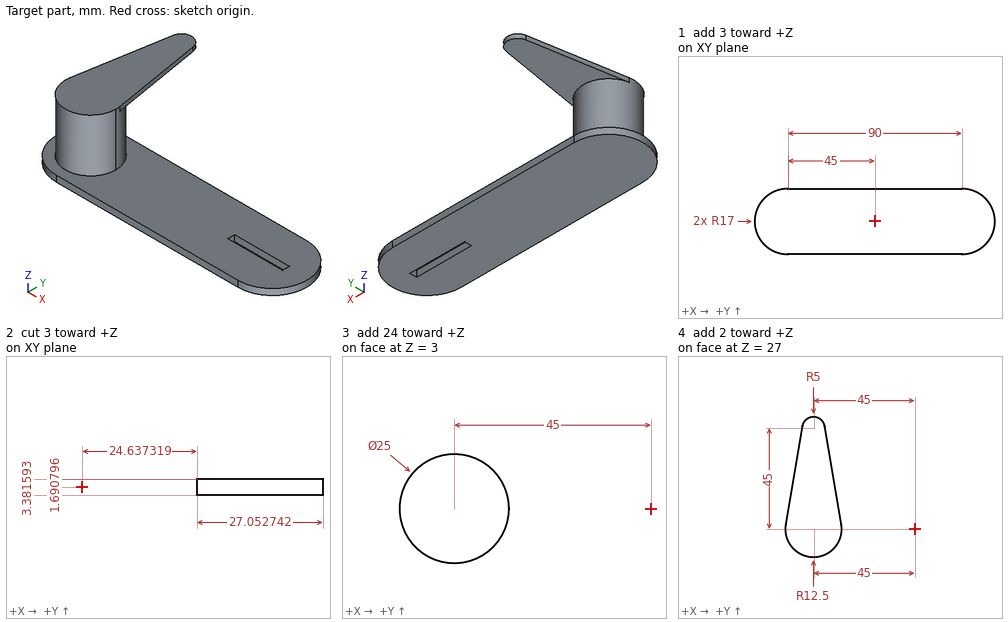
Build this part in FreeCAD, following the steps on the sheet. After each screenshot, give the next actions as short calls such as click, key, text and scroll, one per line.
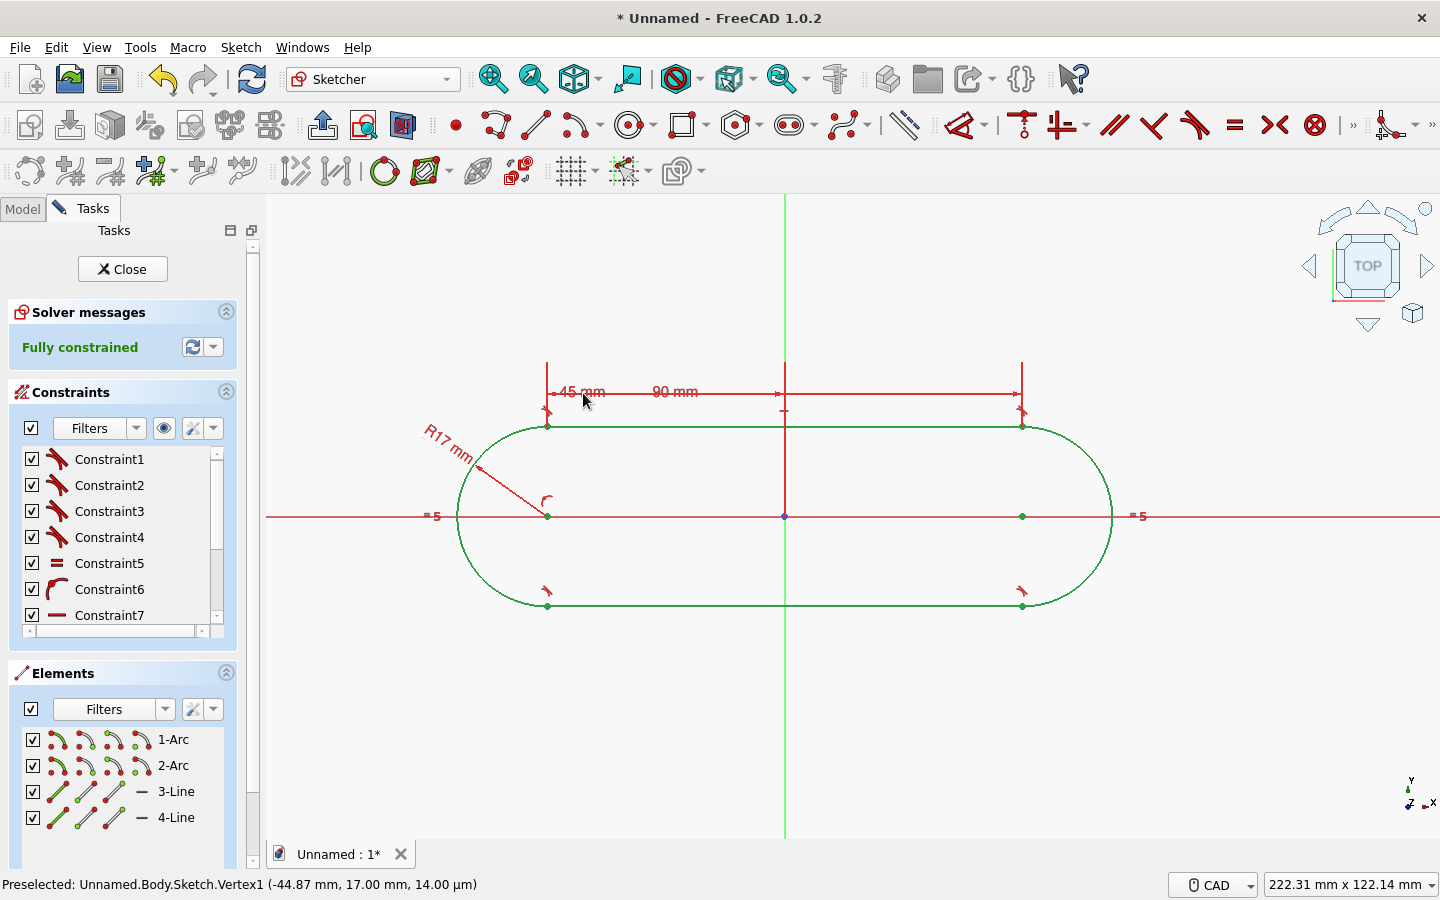
click(123, 269)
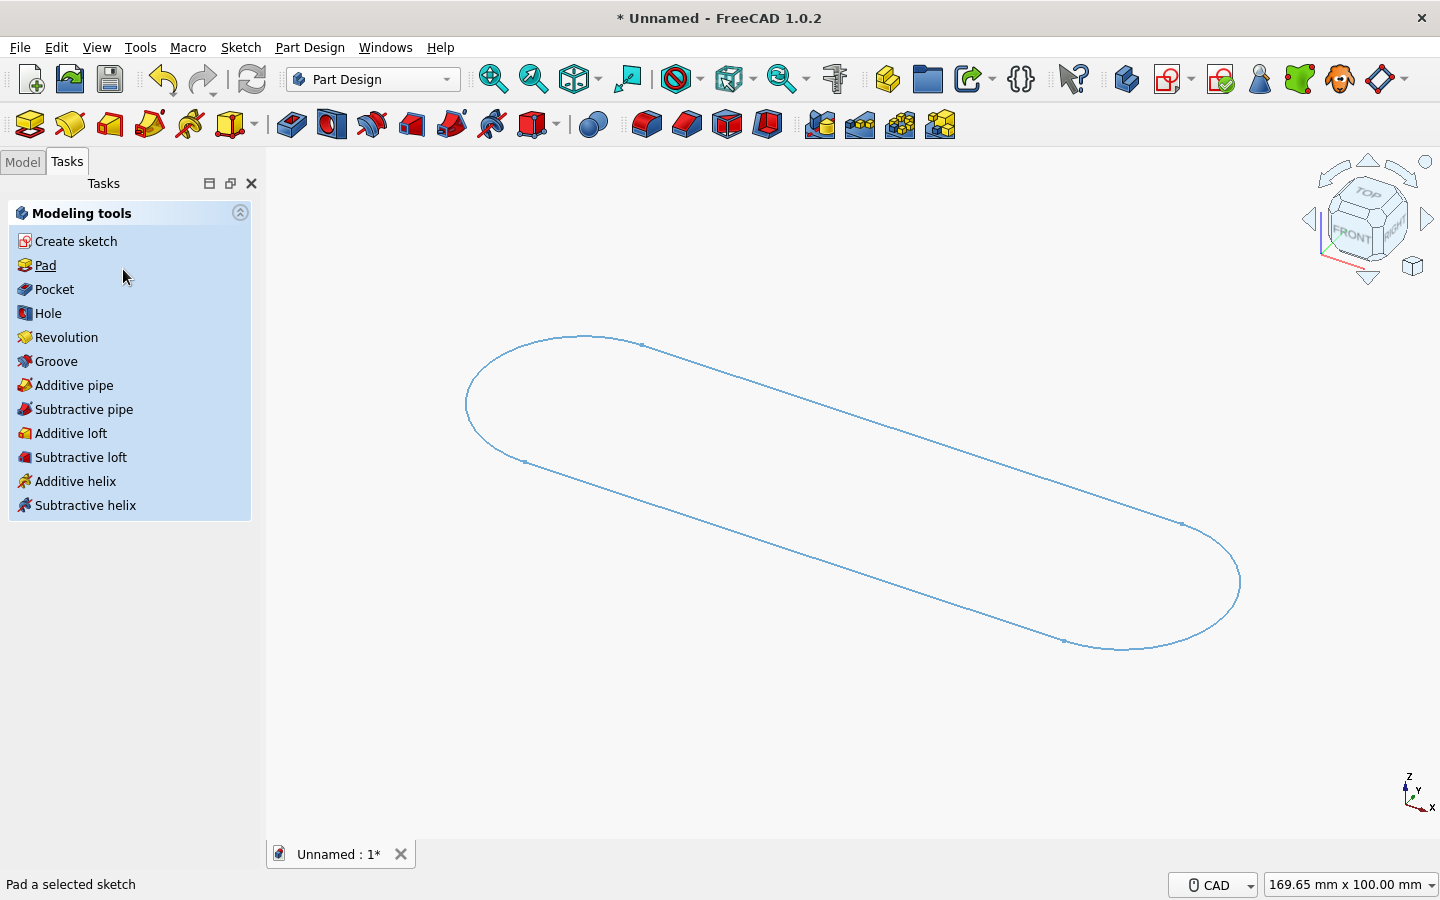
click(30, 124)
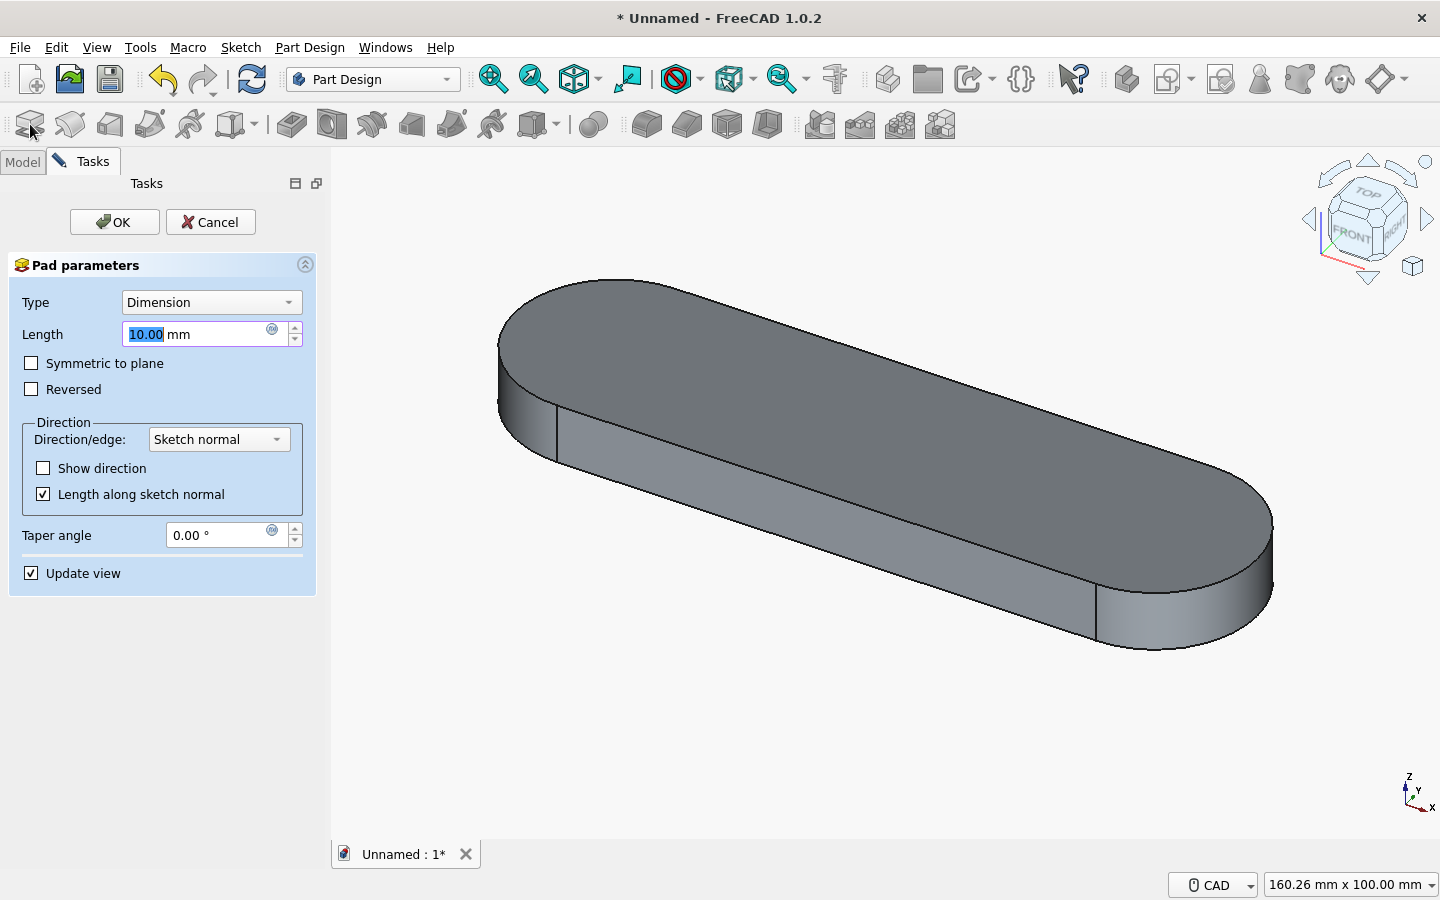
text(3)
key(Tab)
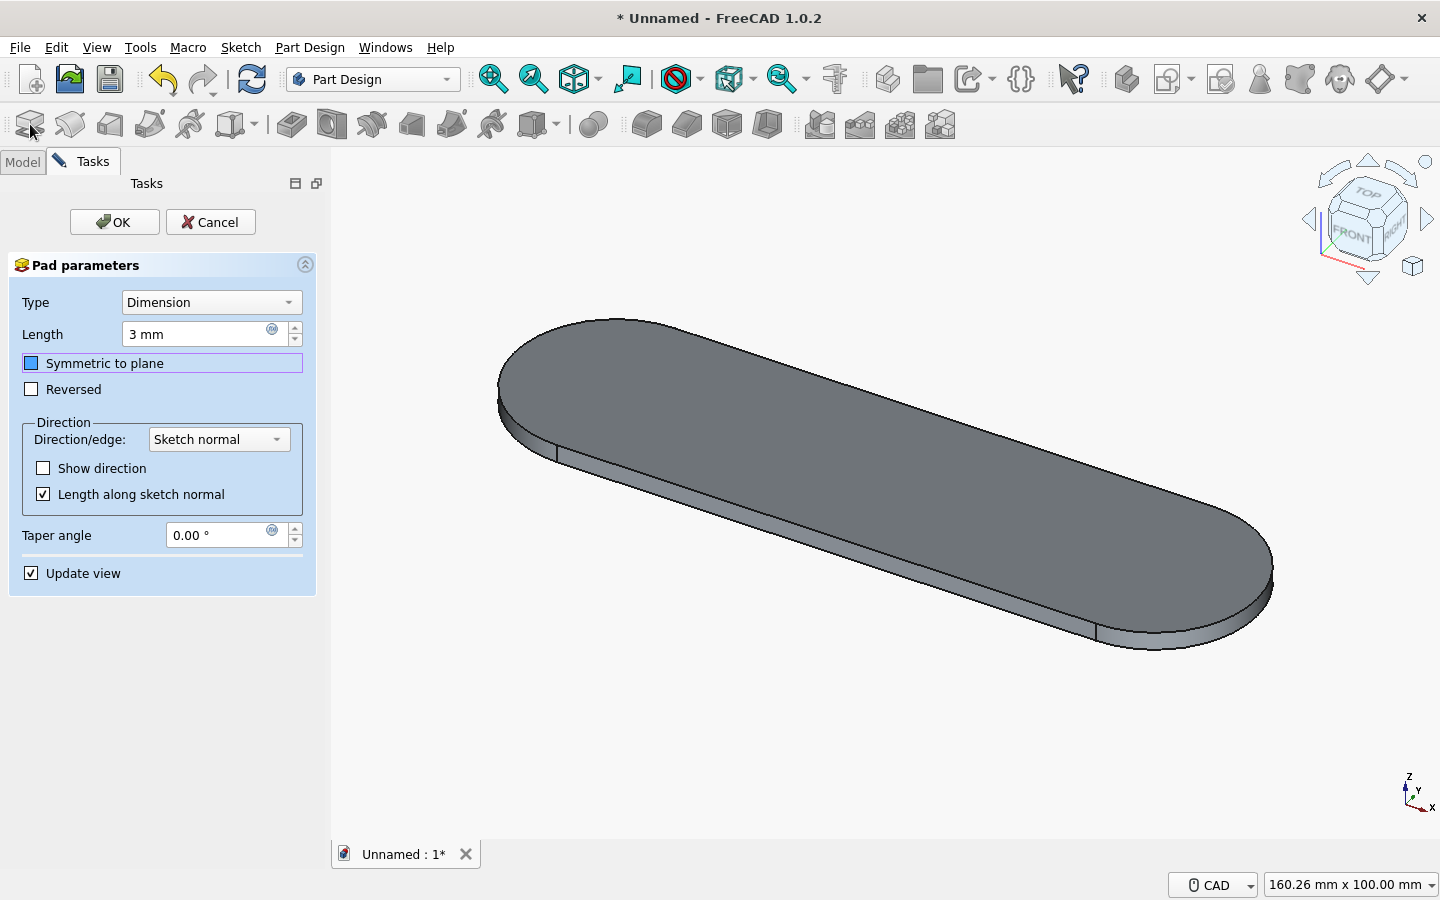
click(115, 222)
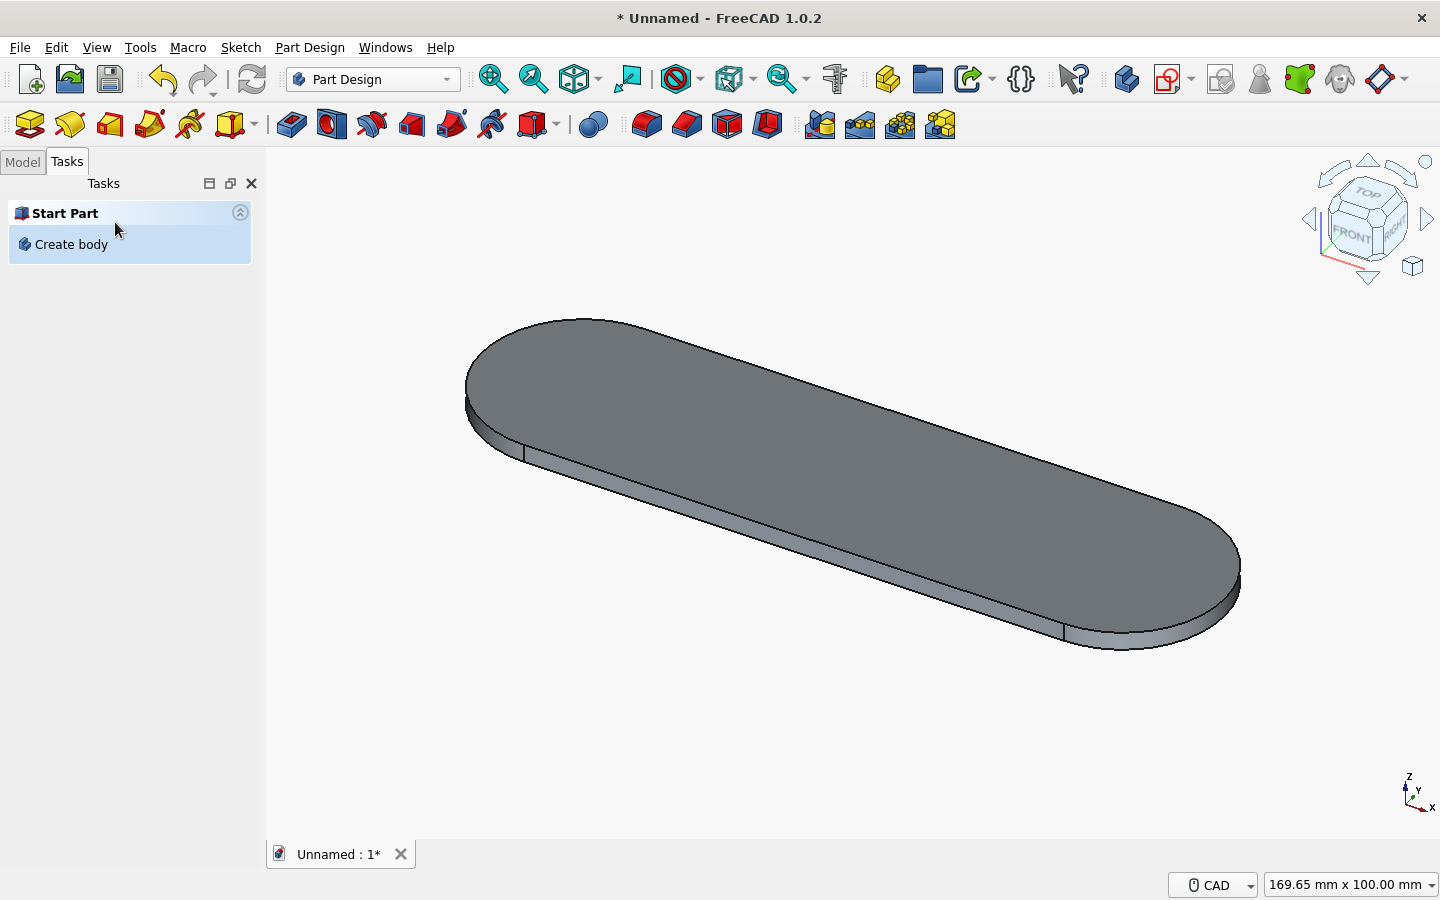
click(1168, 80)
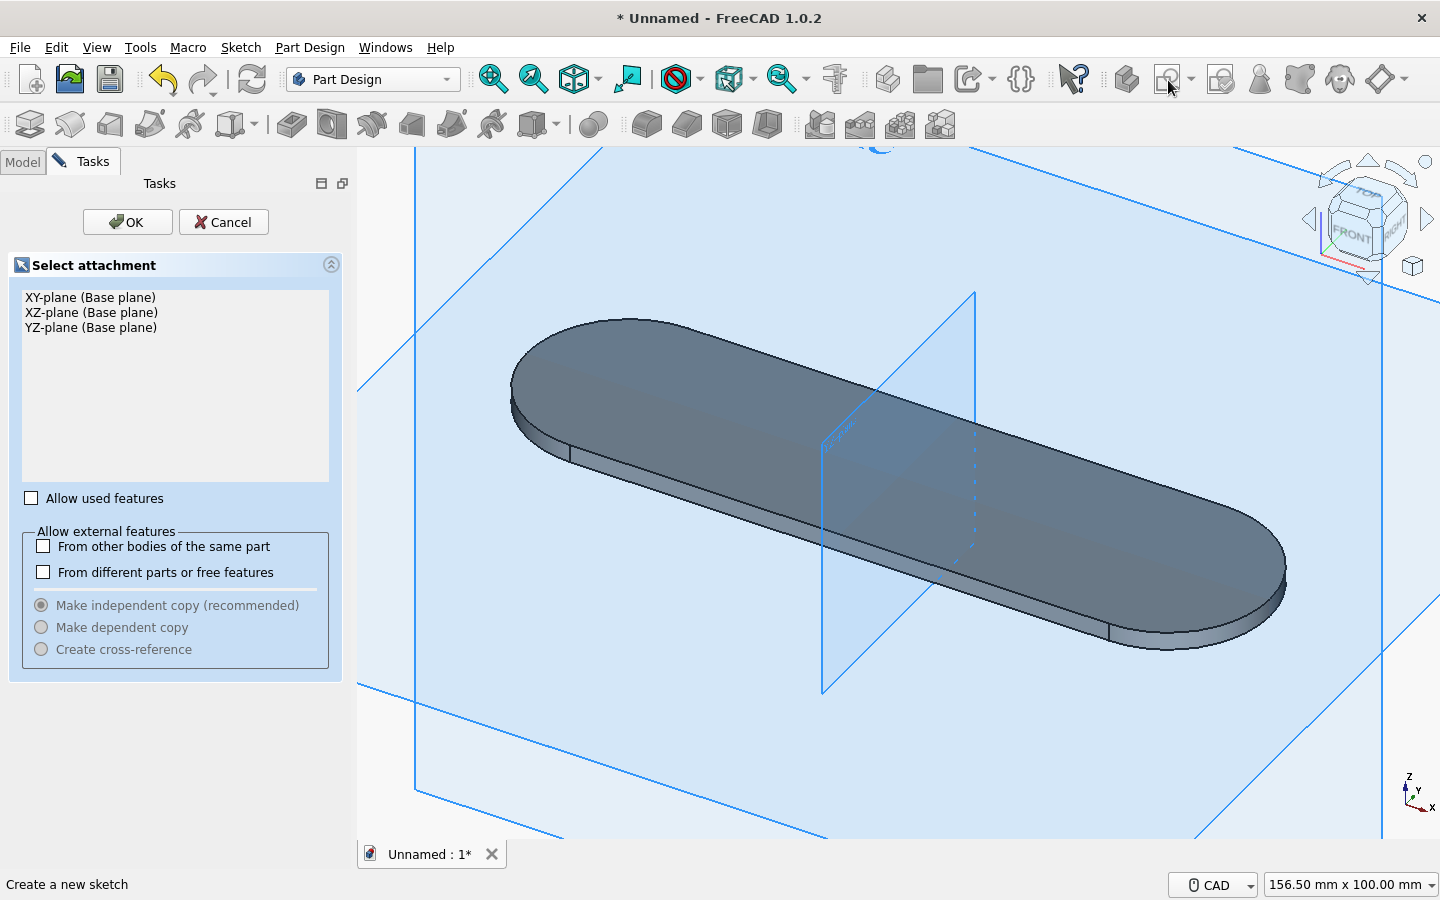
click(82, 298)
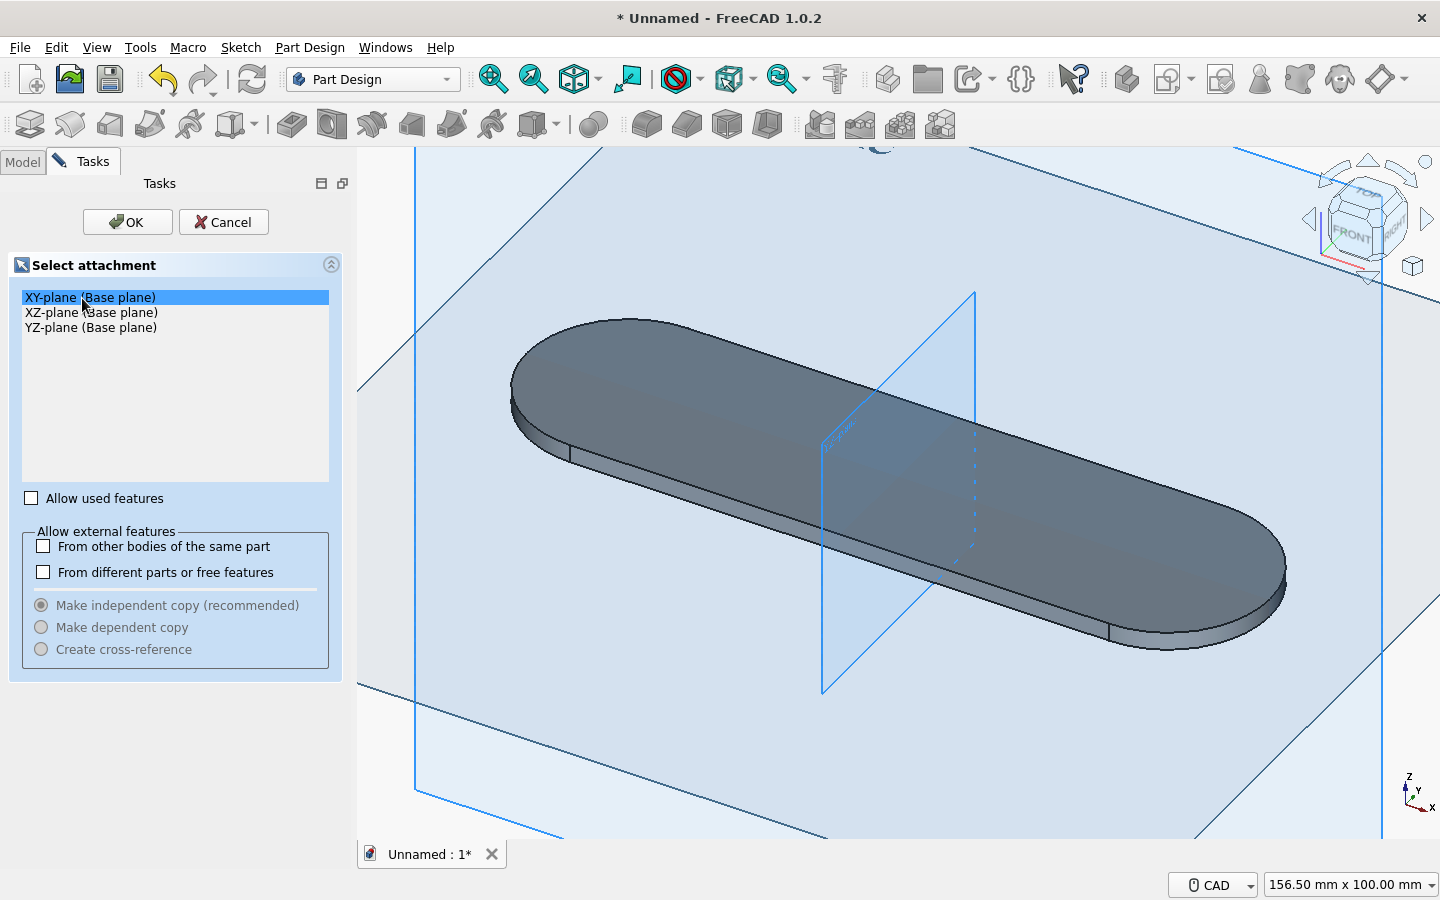
click(128, 222)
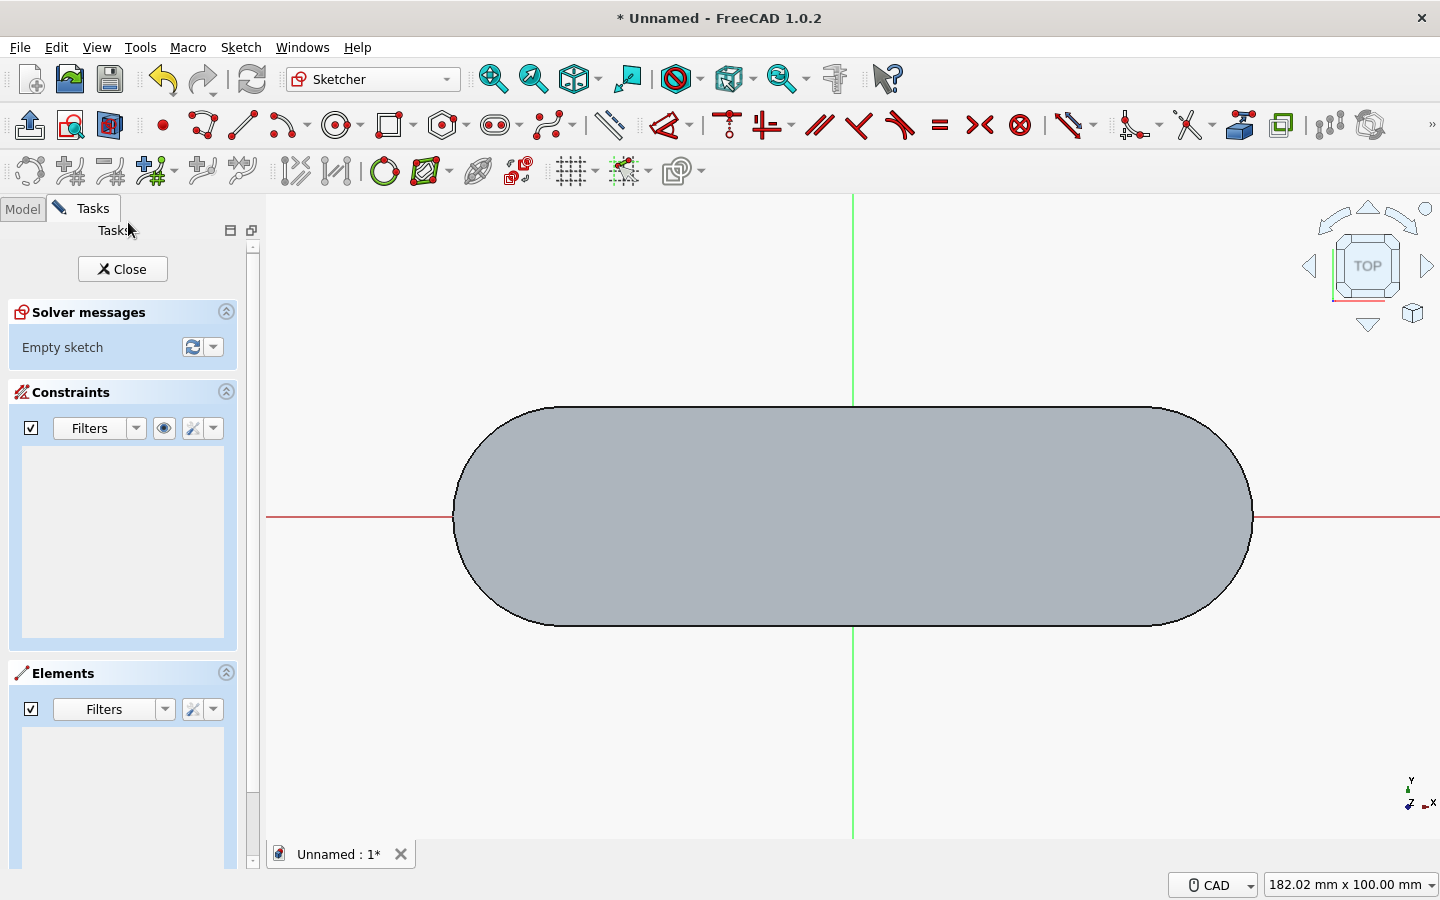
key(q)
key(s)